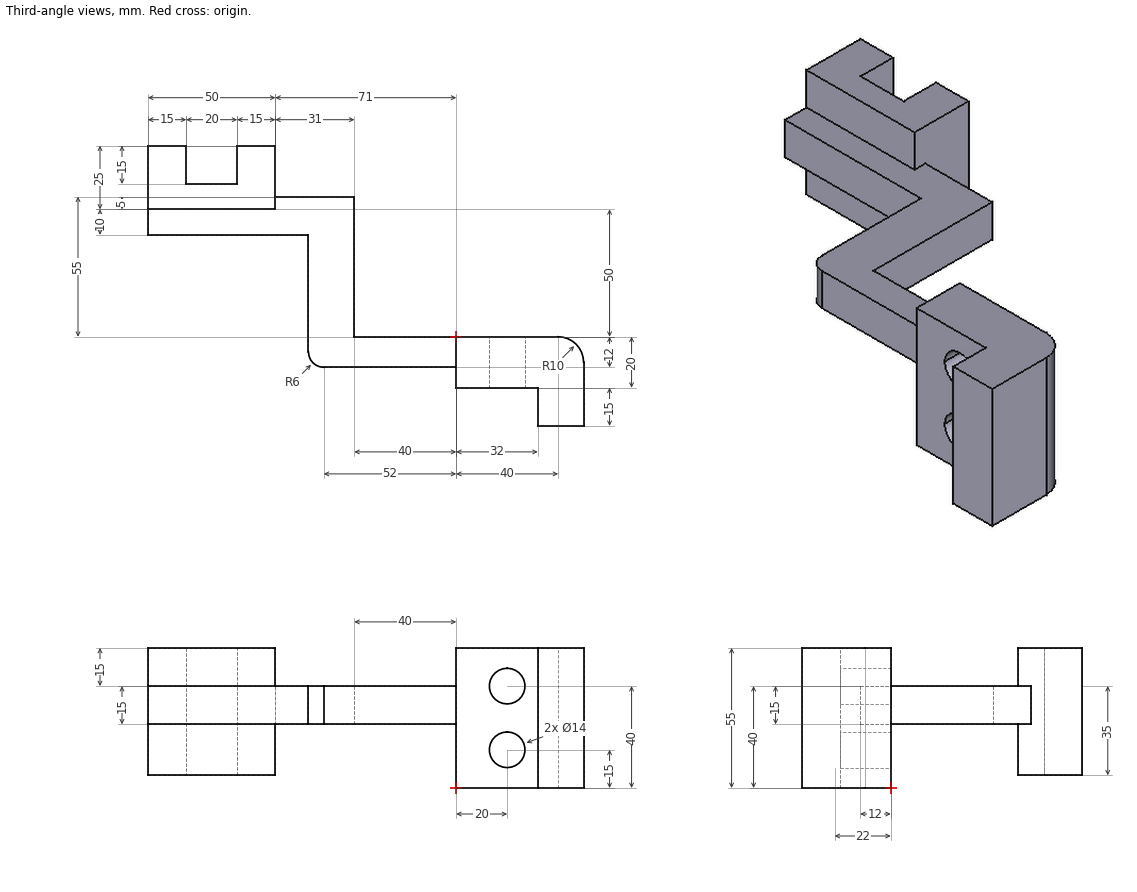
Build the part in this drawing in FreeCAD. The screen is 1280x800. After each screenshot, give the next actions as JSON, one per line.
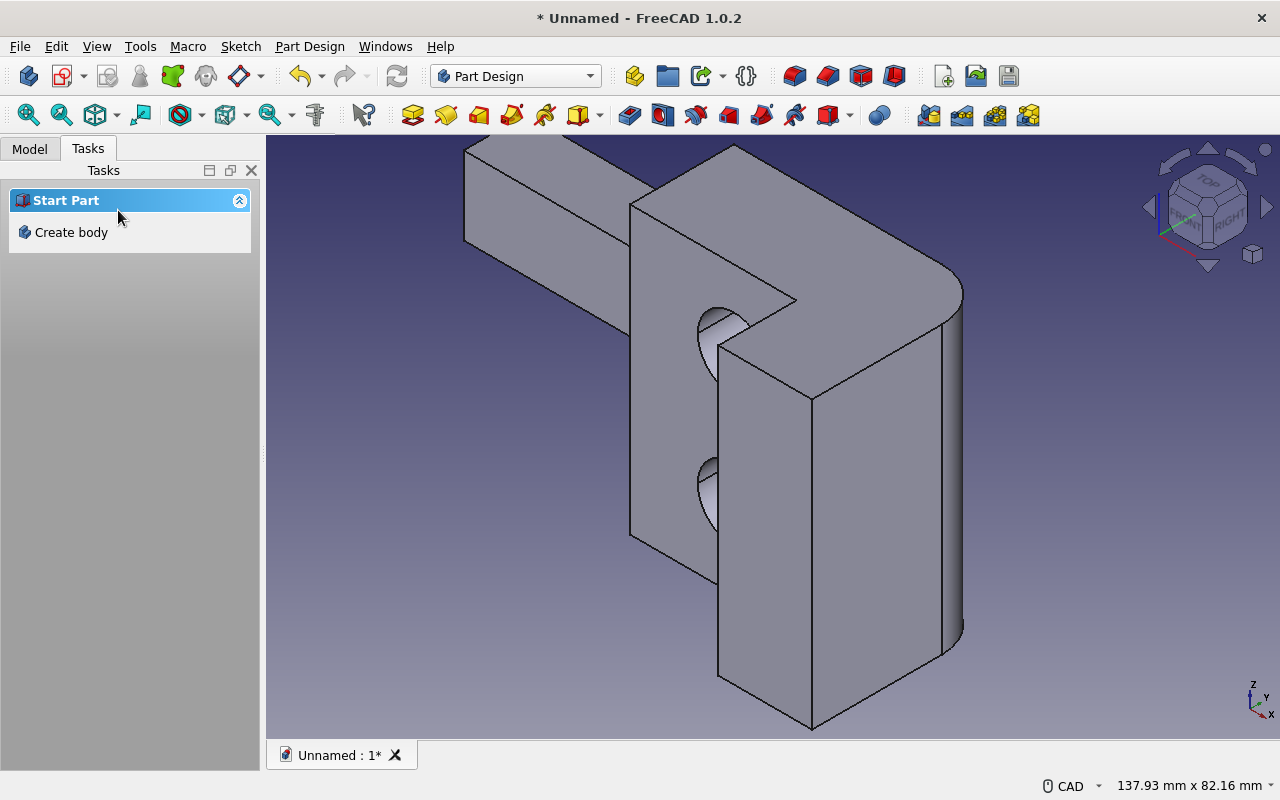
{"action": "left_click", "coordinate": [29, 116]}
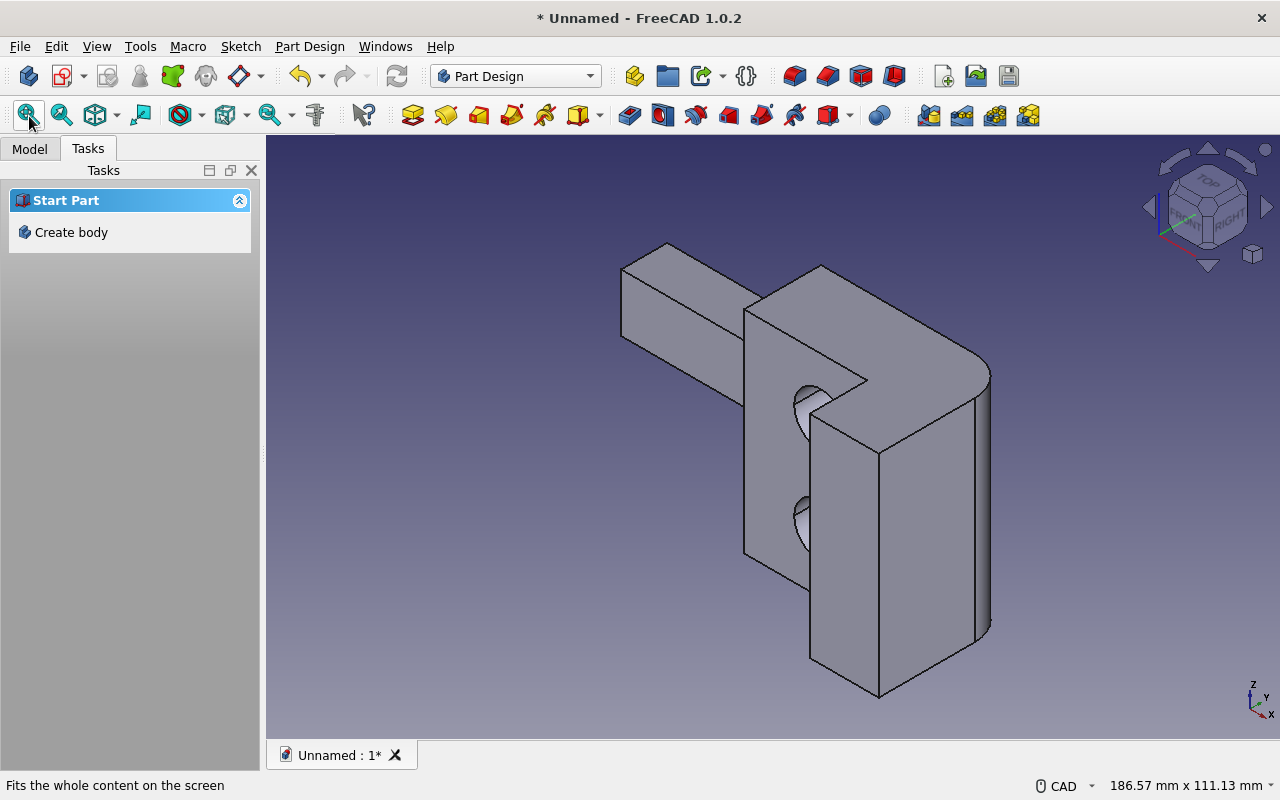
{"action": "left_click", "coordinate": [721, 300]}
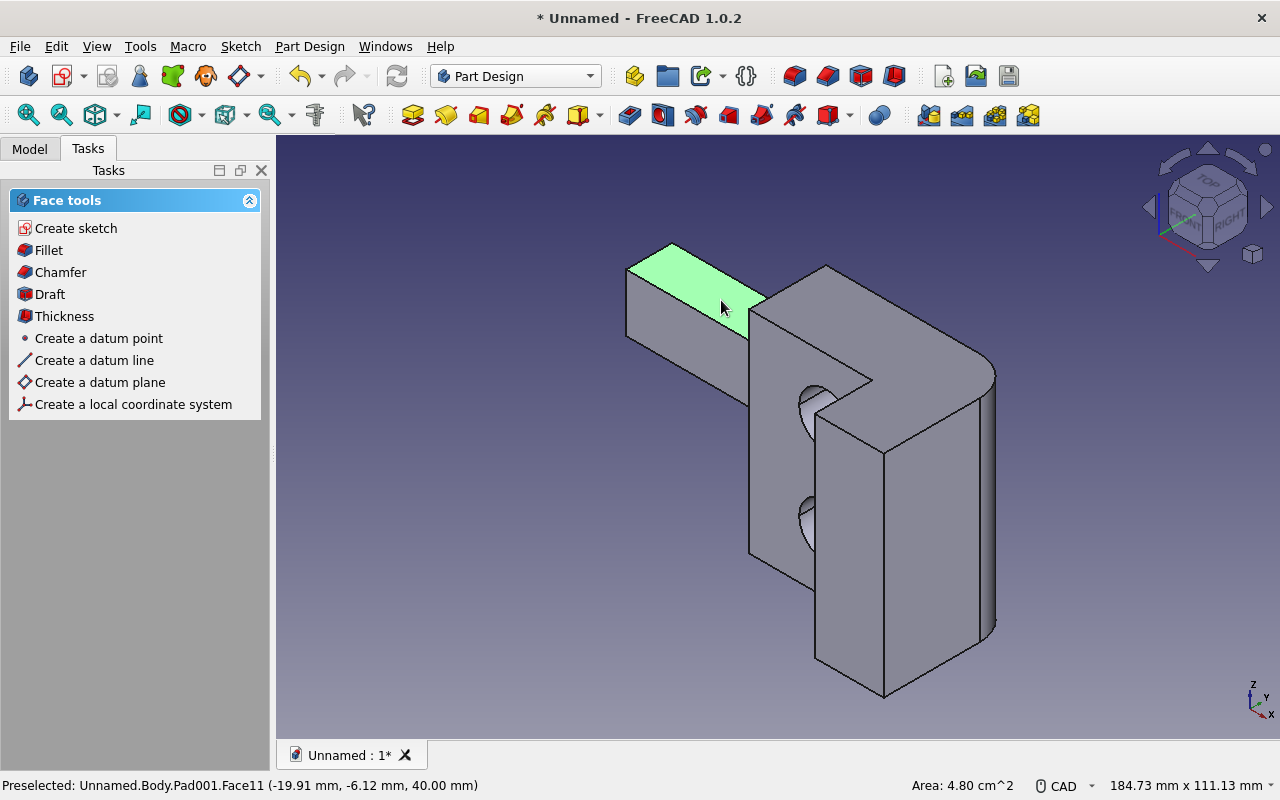
{"action": "left_click", "coordinate": [62, 76]}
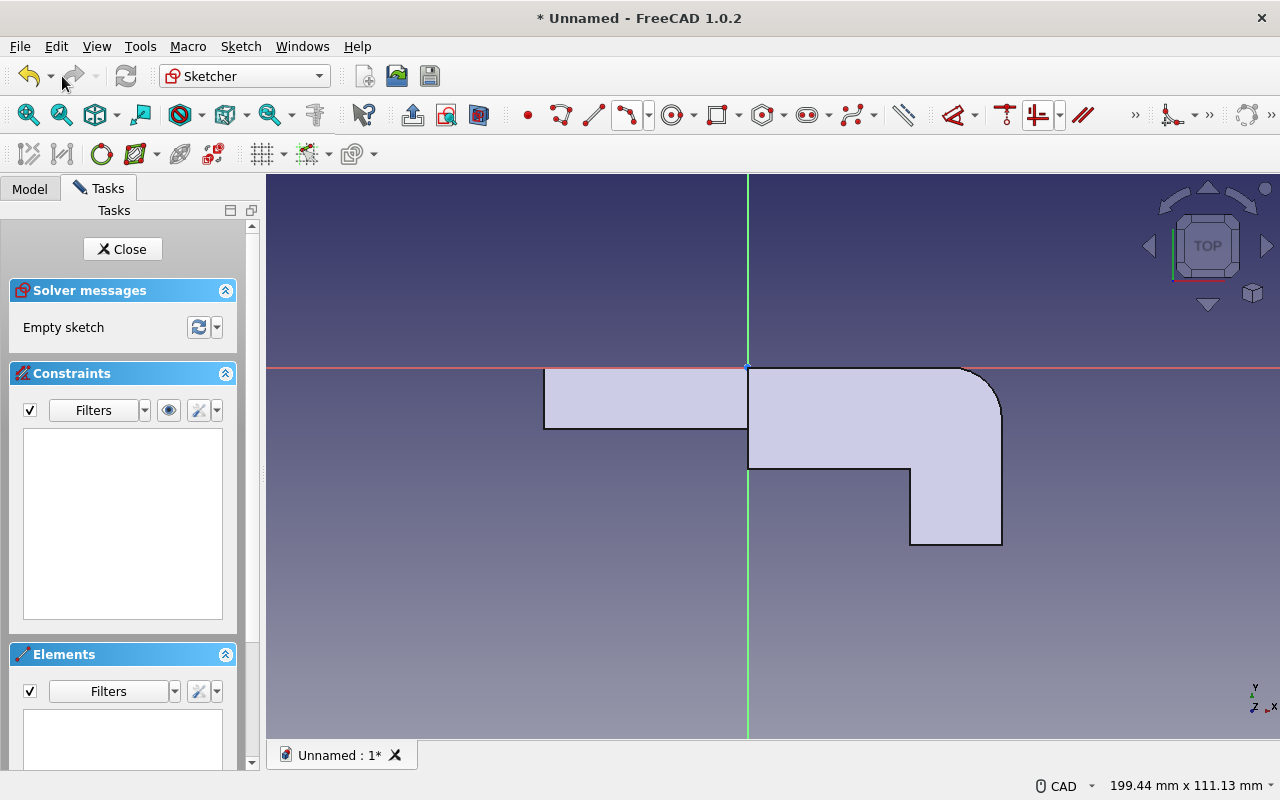
{"action": "scroll", "coordinate": [1115, 711], "scroll_direction": "down", "scroll_amount": 2}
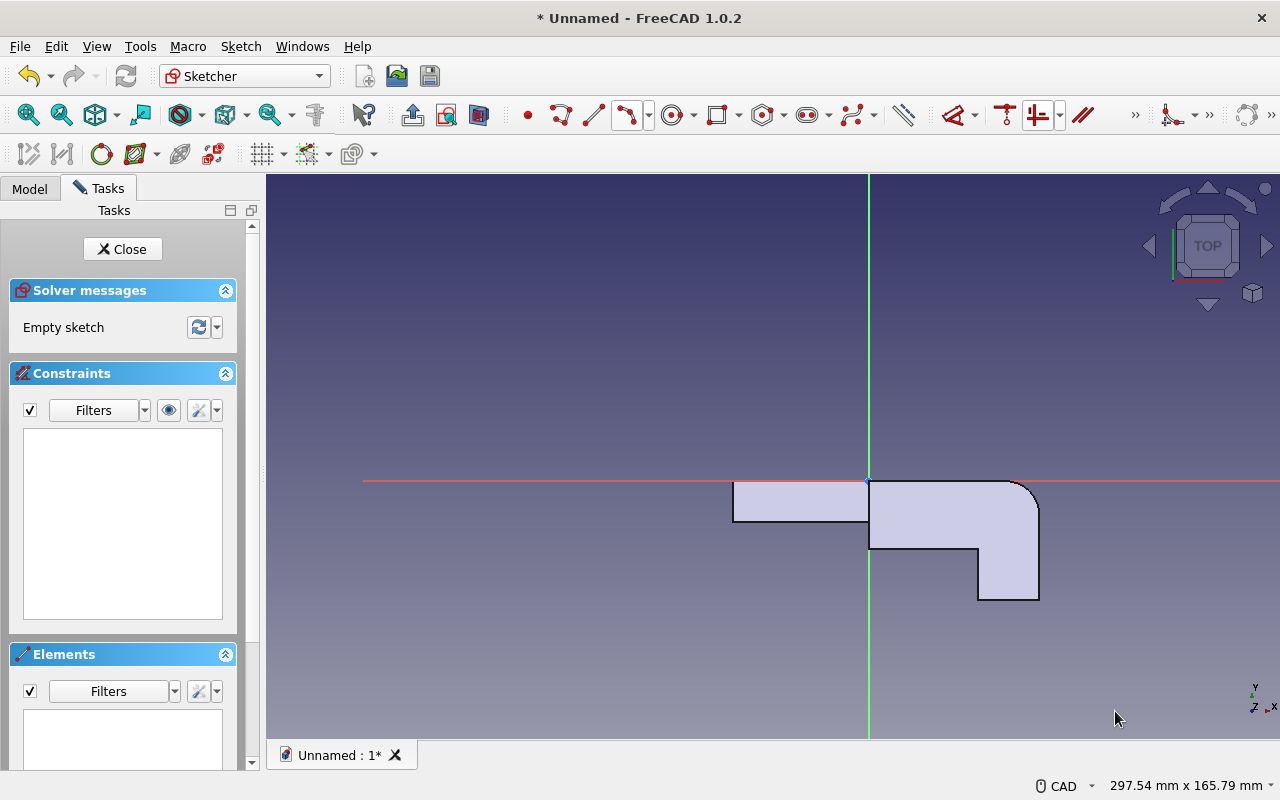
{"action": "scroll", "coordinate": [578, 309], "scroll_direction": "up", "scroll_amount": 2}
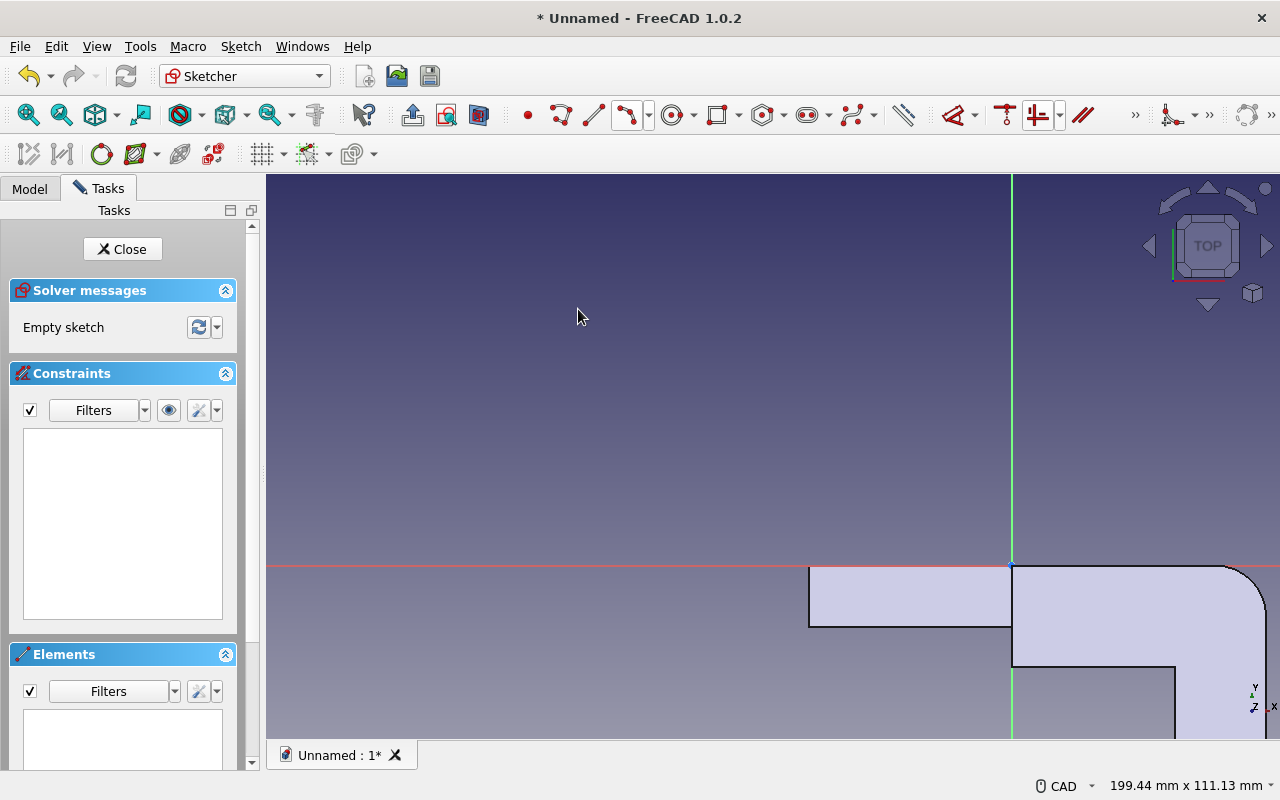
{"action": "left_click", "coordinate": [561, 116]}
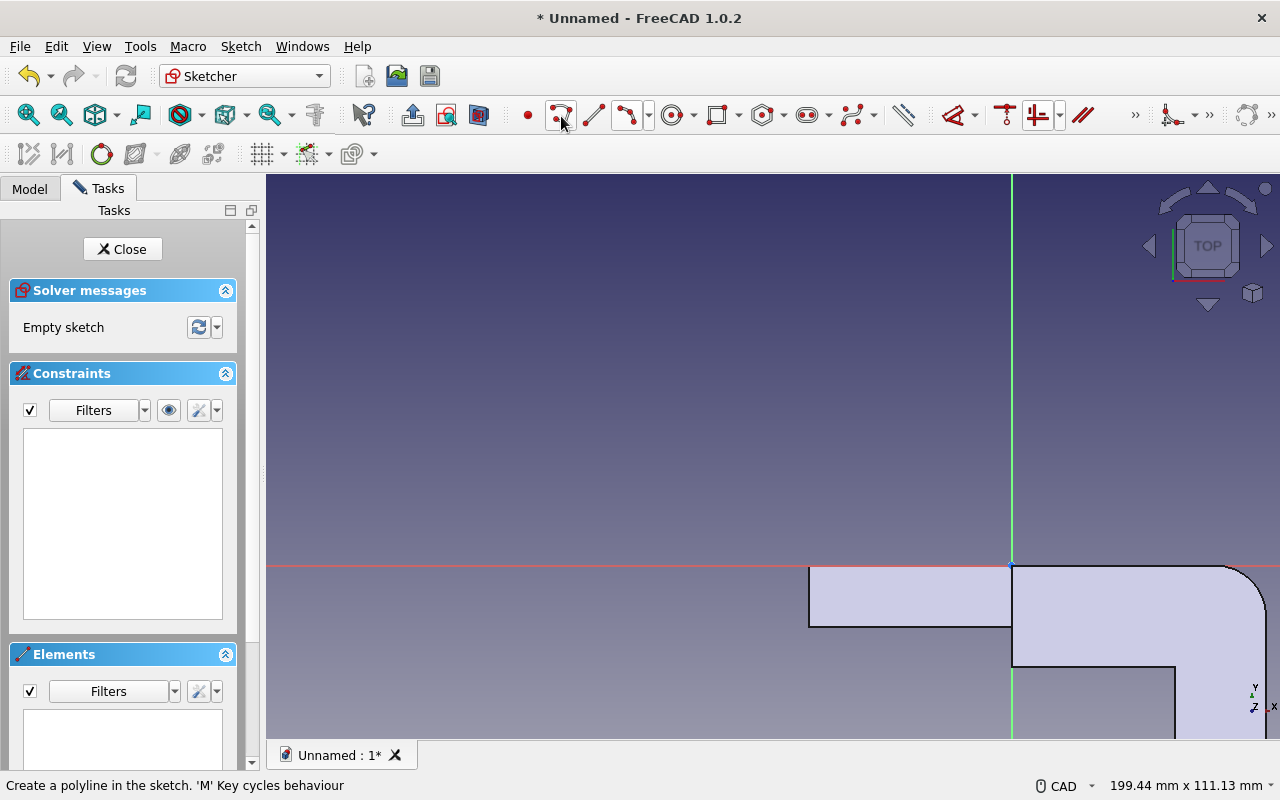
{"action": "left_click", "coordinate": [748, 627]}
{"action": "left_click", "coordinate": [1012, 627]}
{"action": "left_click", "coordinate": [1012, 566]}
{"action": "left_click", "coordinate": [809, 557]}
{"action": "left_click", "coordinate": [809, 286]}
{"action": "left_click", "coordinate": [651, 286]}
{"action": "left_click", "coordinate": [651, 311]}
{"action": "left_click", "coordinate": [397, 311]}
{"action": "left_click", "coordinate": [397, 362]}
{"action": "left_click", "coordinate": [717, 362]}
{"action": "left_click", "coordinate": [717, 596]}
{"action": "right_click", "coordinate": [717, 596]}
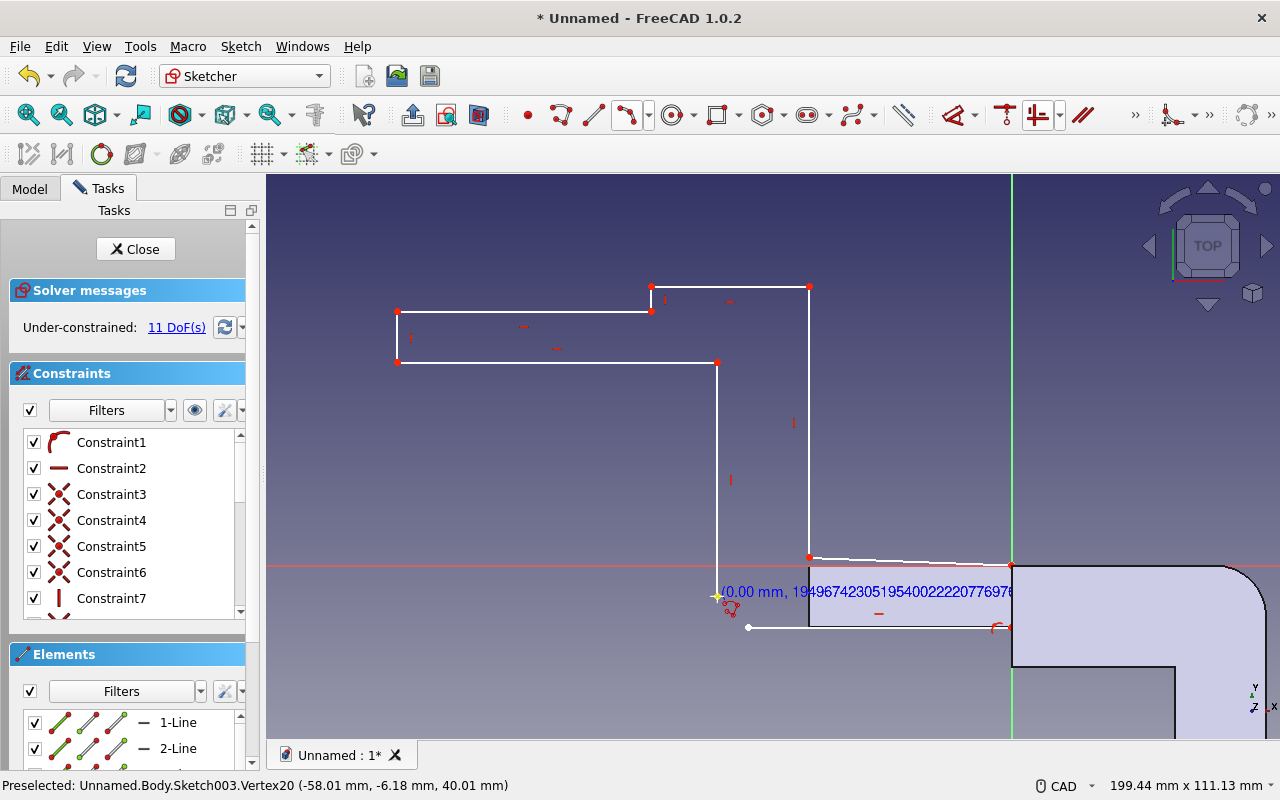
{"action": "left_click", "coordinate": [626, 116]}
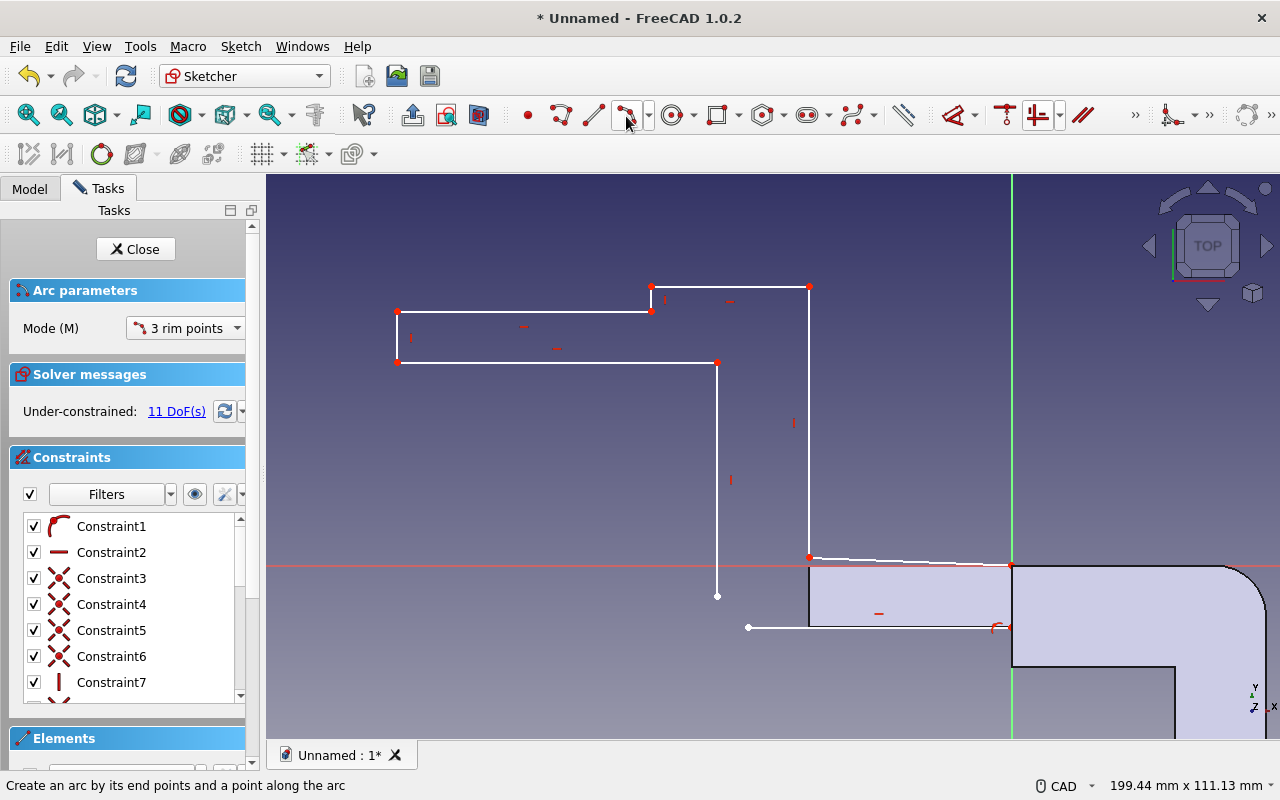
{"action": "left_click", "coordinate": [717, 597]}
{"action": "left_click", "coordinate": [748, 628]}